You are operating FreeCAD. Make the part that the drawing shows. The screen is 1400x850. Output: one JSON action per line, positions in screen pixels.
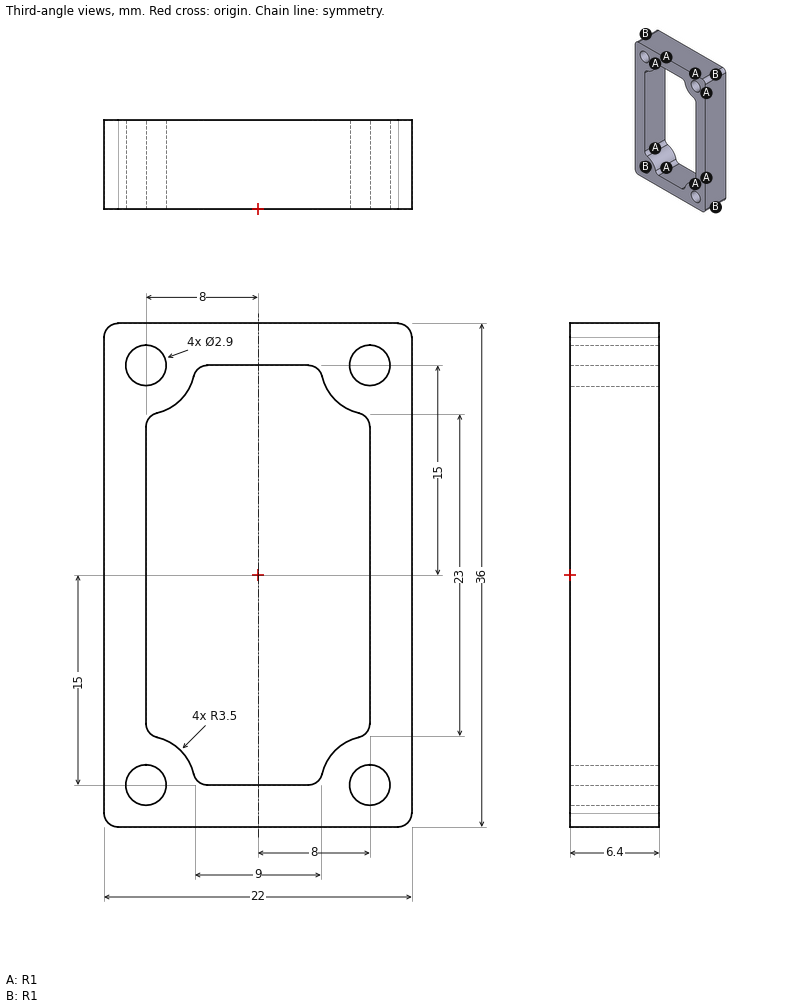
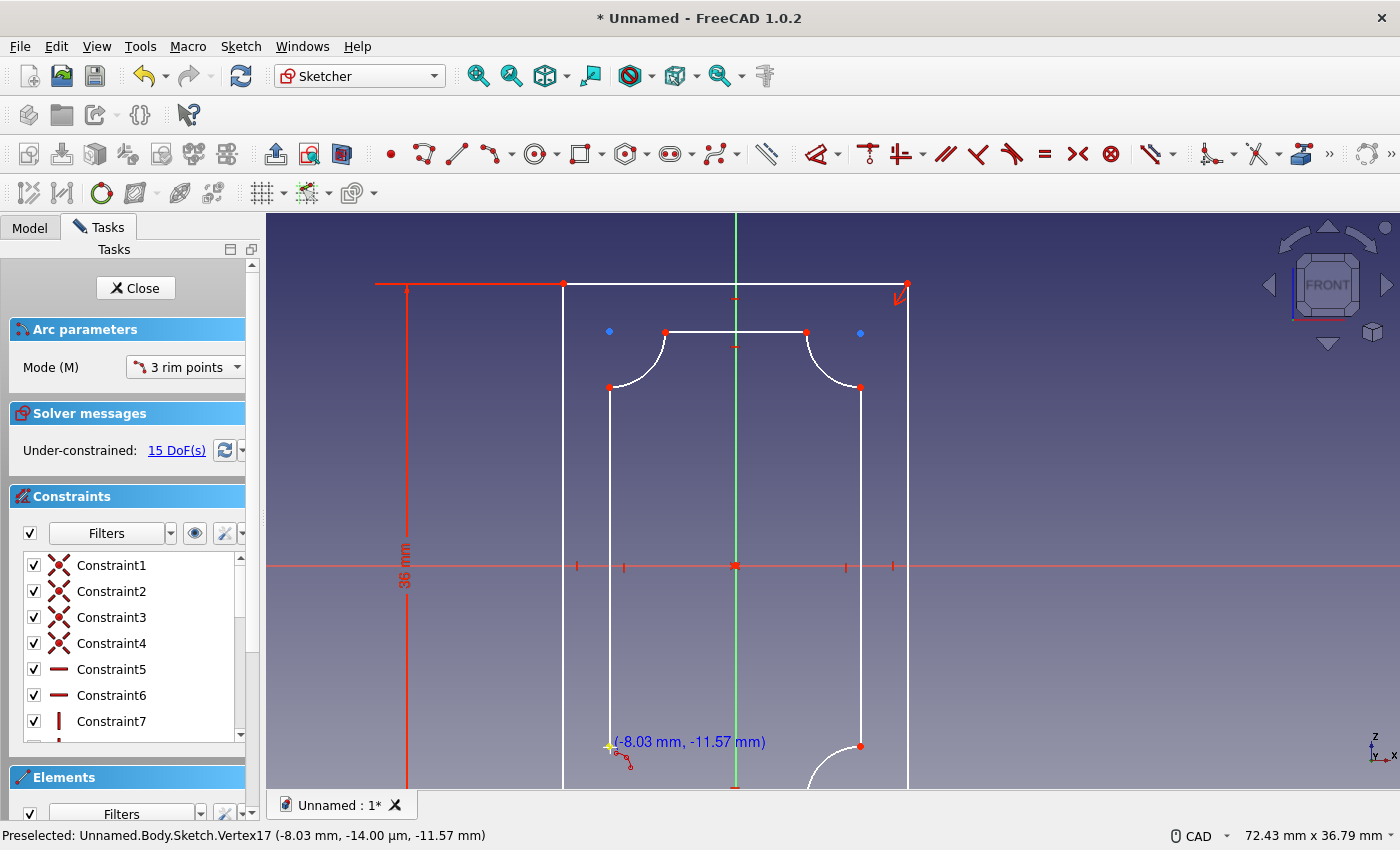
{"action": "scroll", "coordinate": [823, 370], "scroll_direction": "down", "scroll_amount": 2}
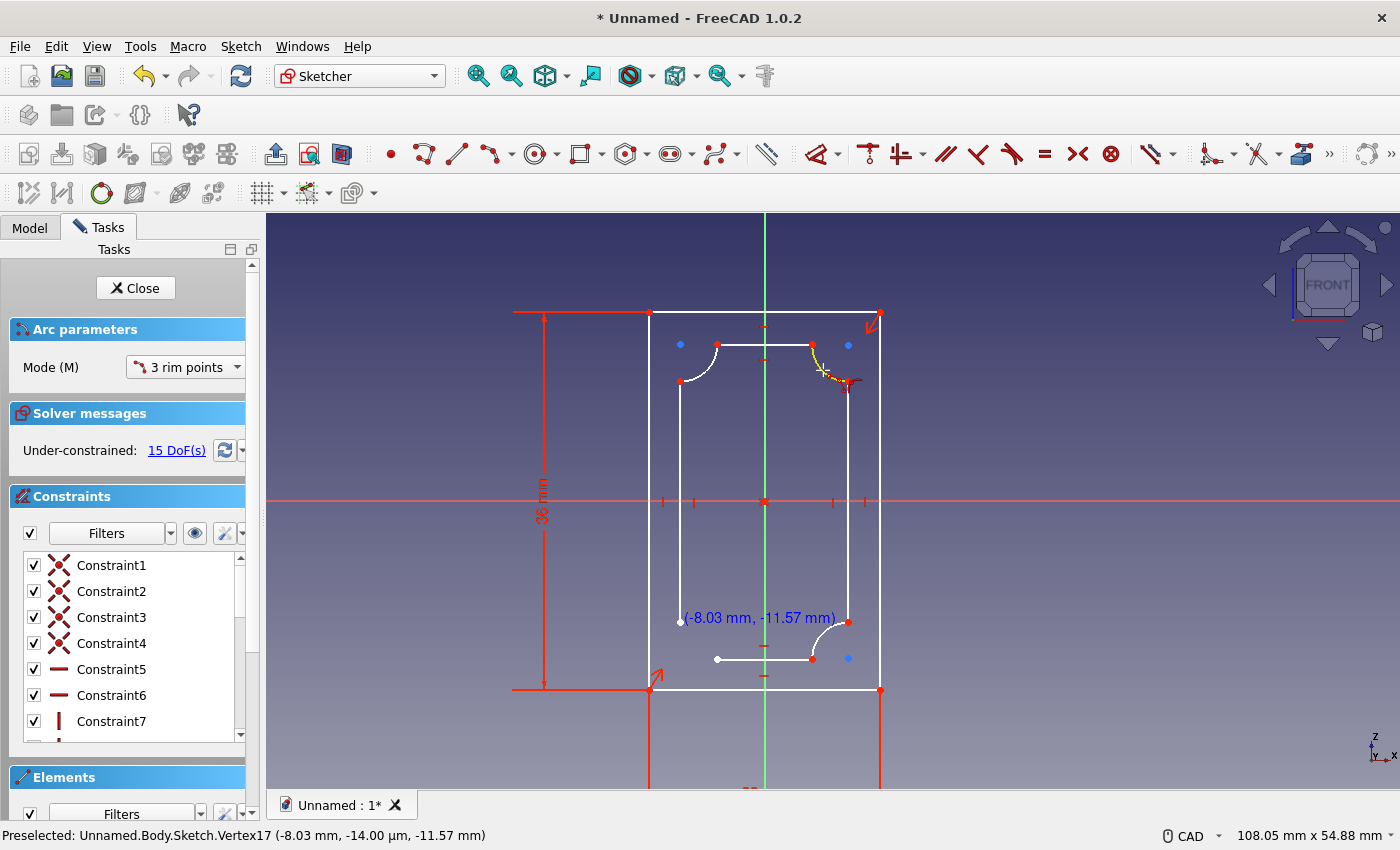
{"action": "left_click", "coordinate": [717, 660]}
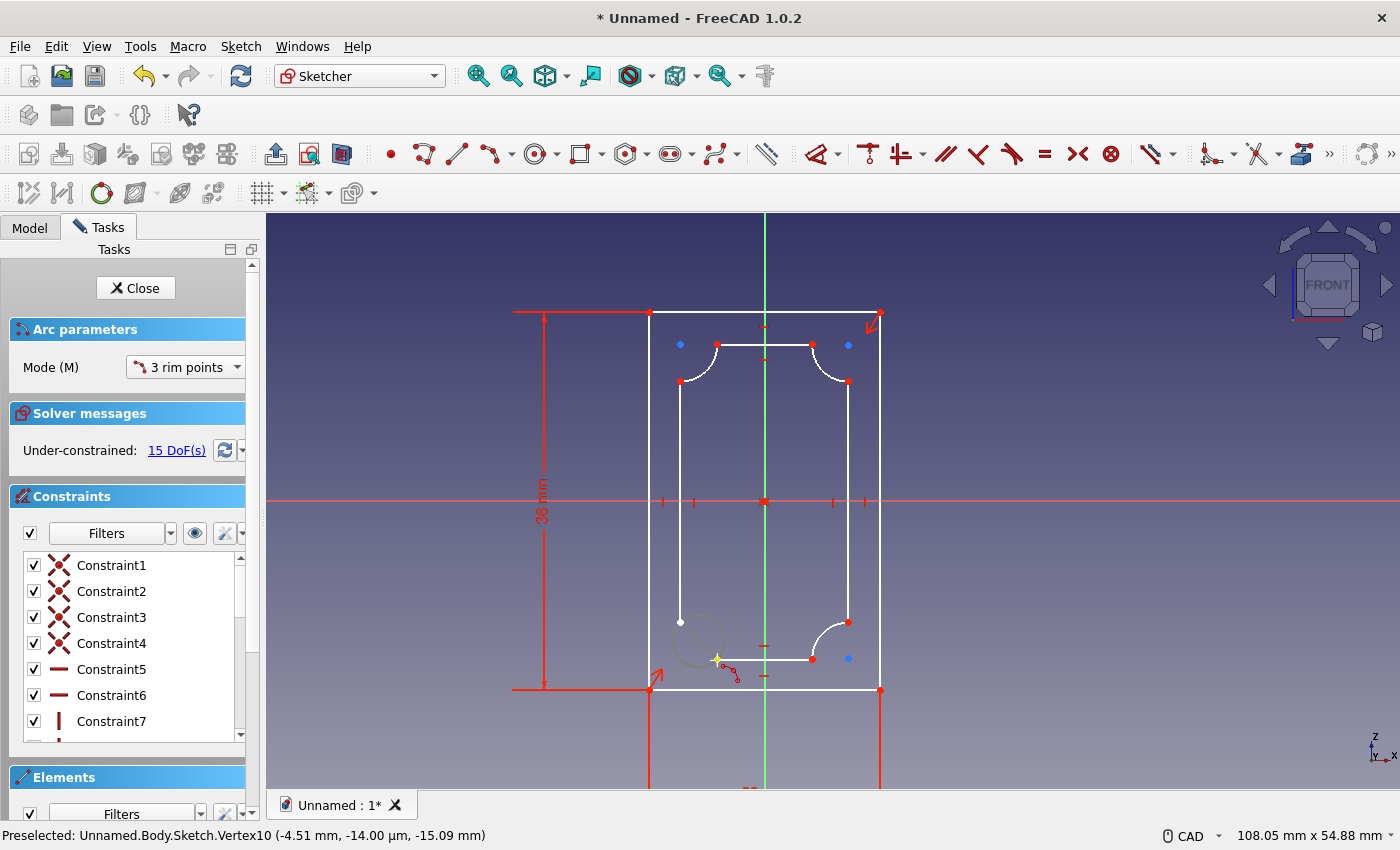
{"action": "scroll", "coordinate": [707, 633], "scroll_direction": "up", "scroll_amount": 2}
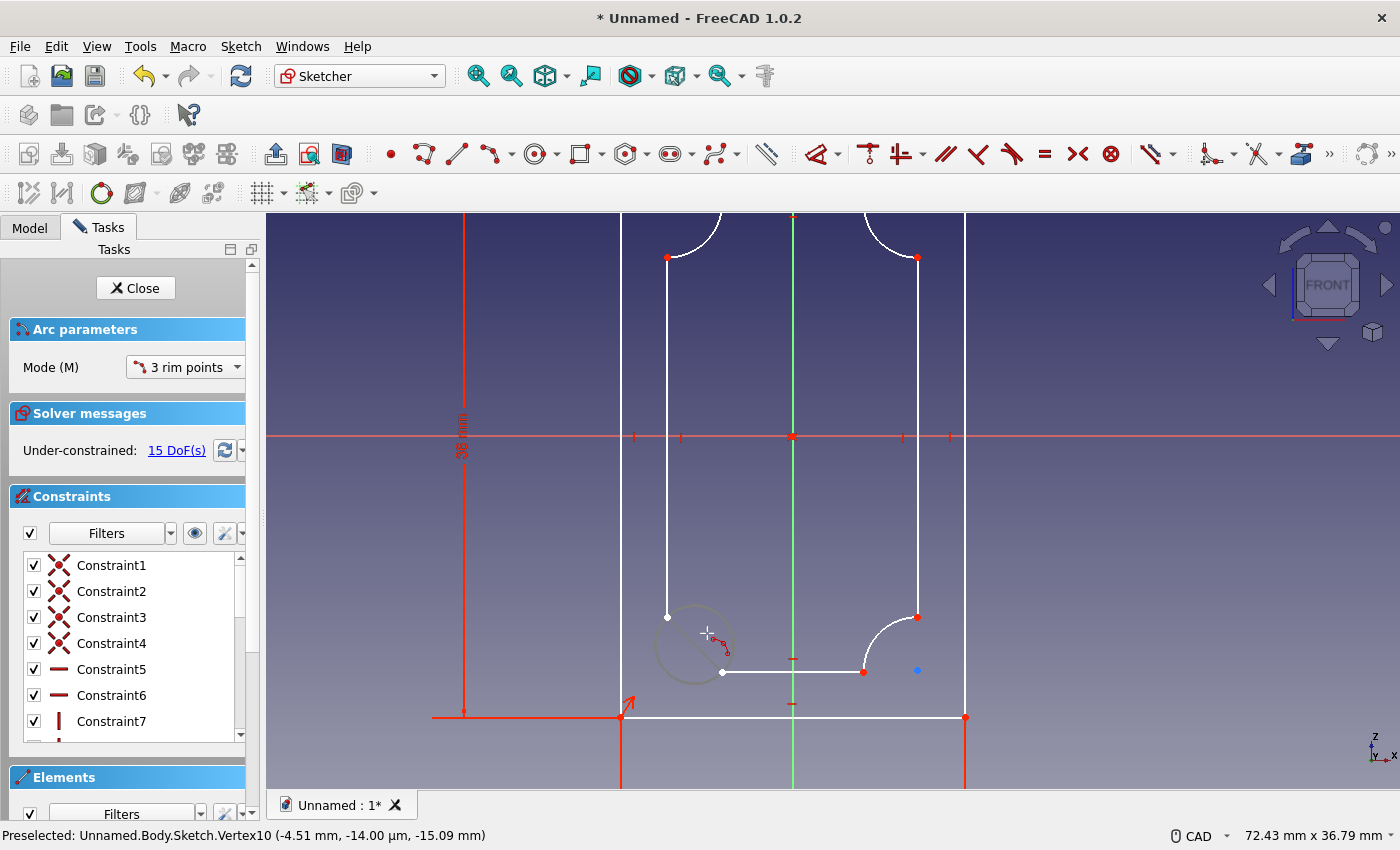
{"action": "left_click", "coordinate": [706, 632]}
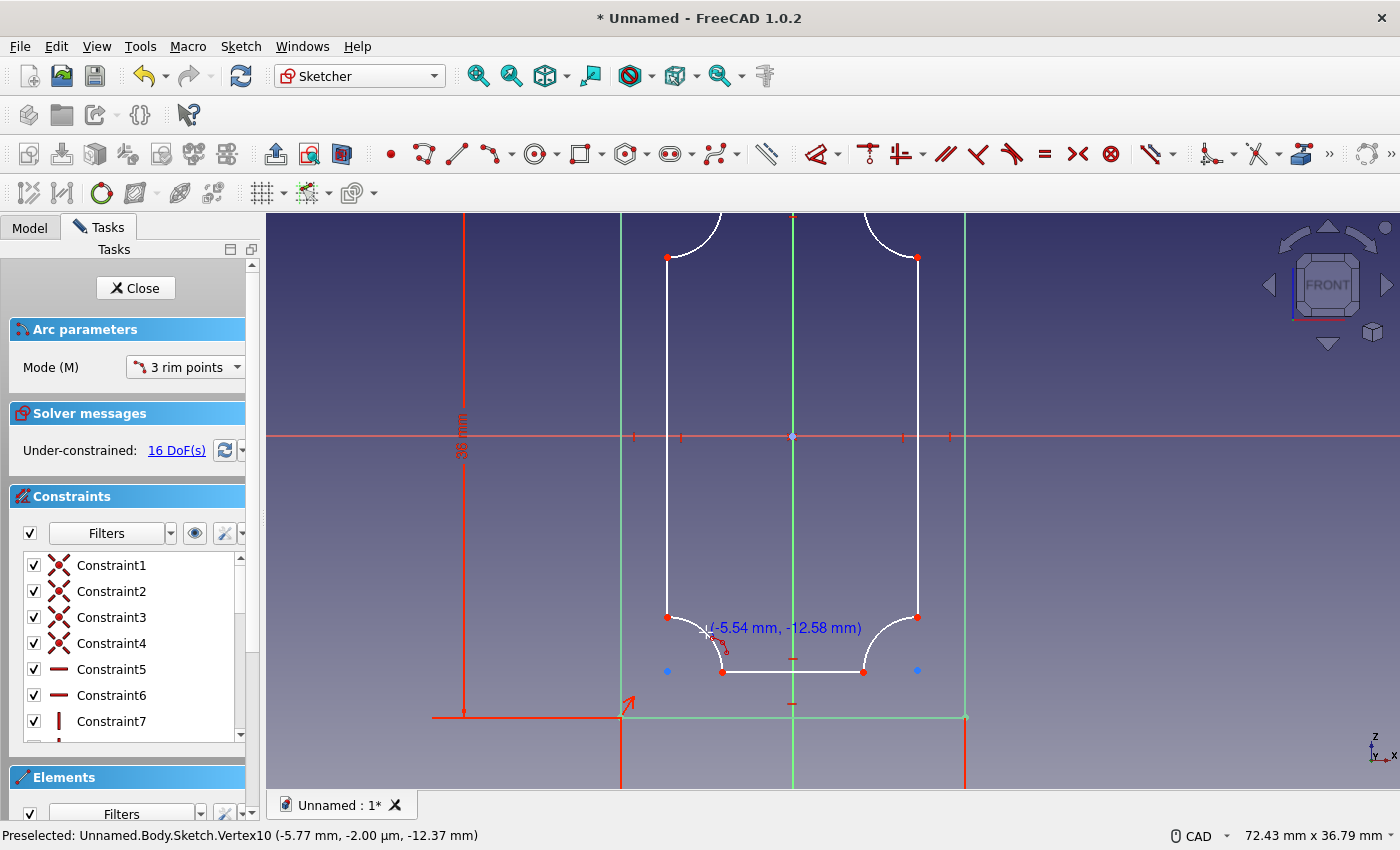
{"action": "left_click", "coordinate": [534, 154]}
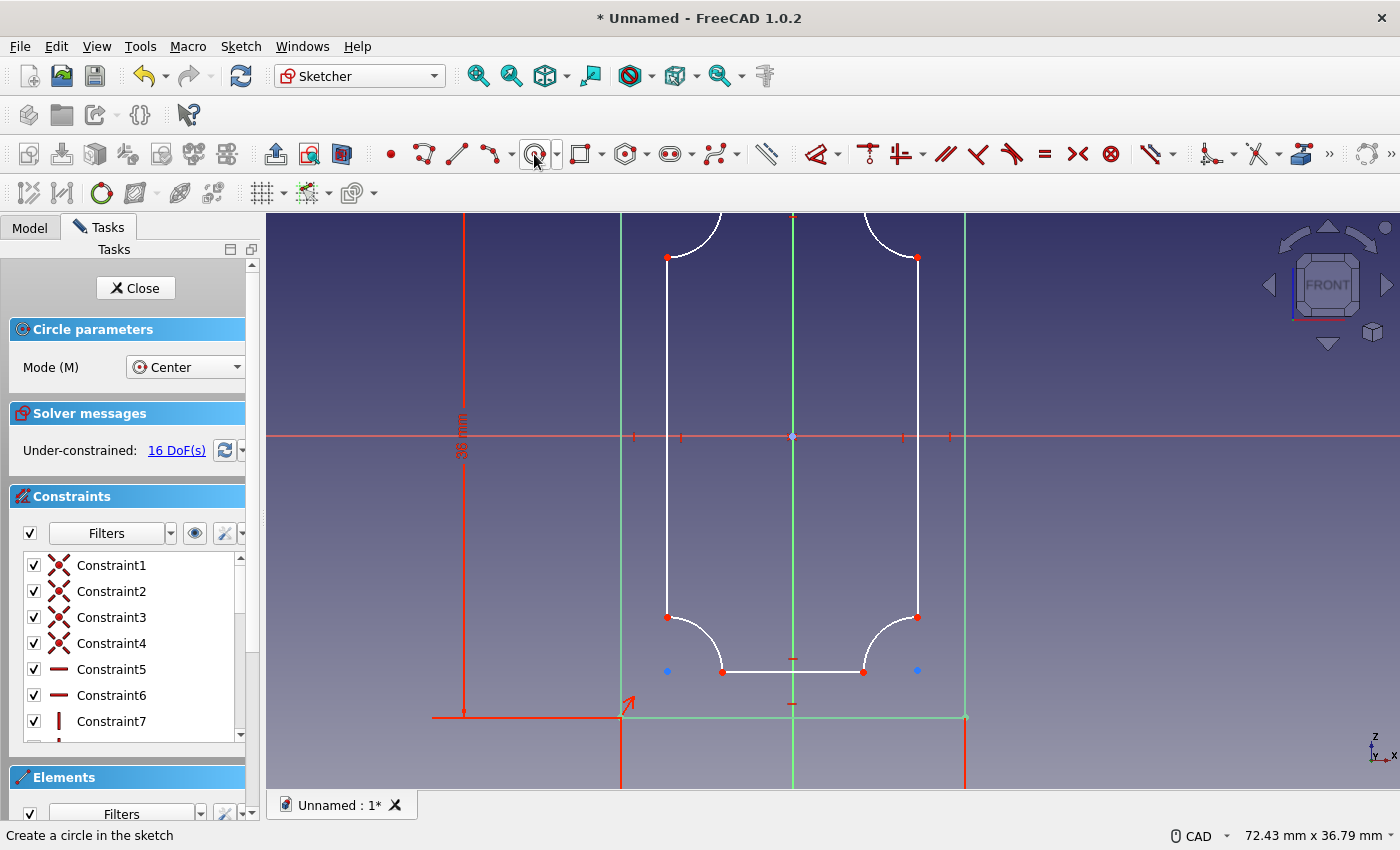
{"action": "scroll", "coordinate": [707, 633], "scroll_direction": "down", "scroll_amount": 2}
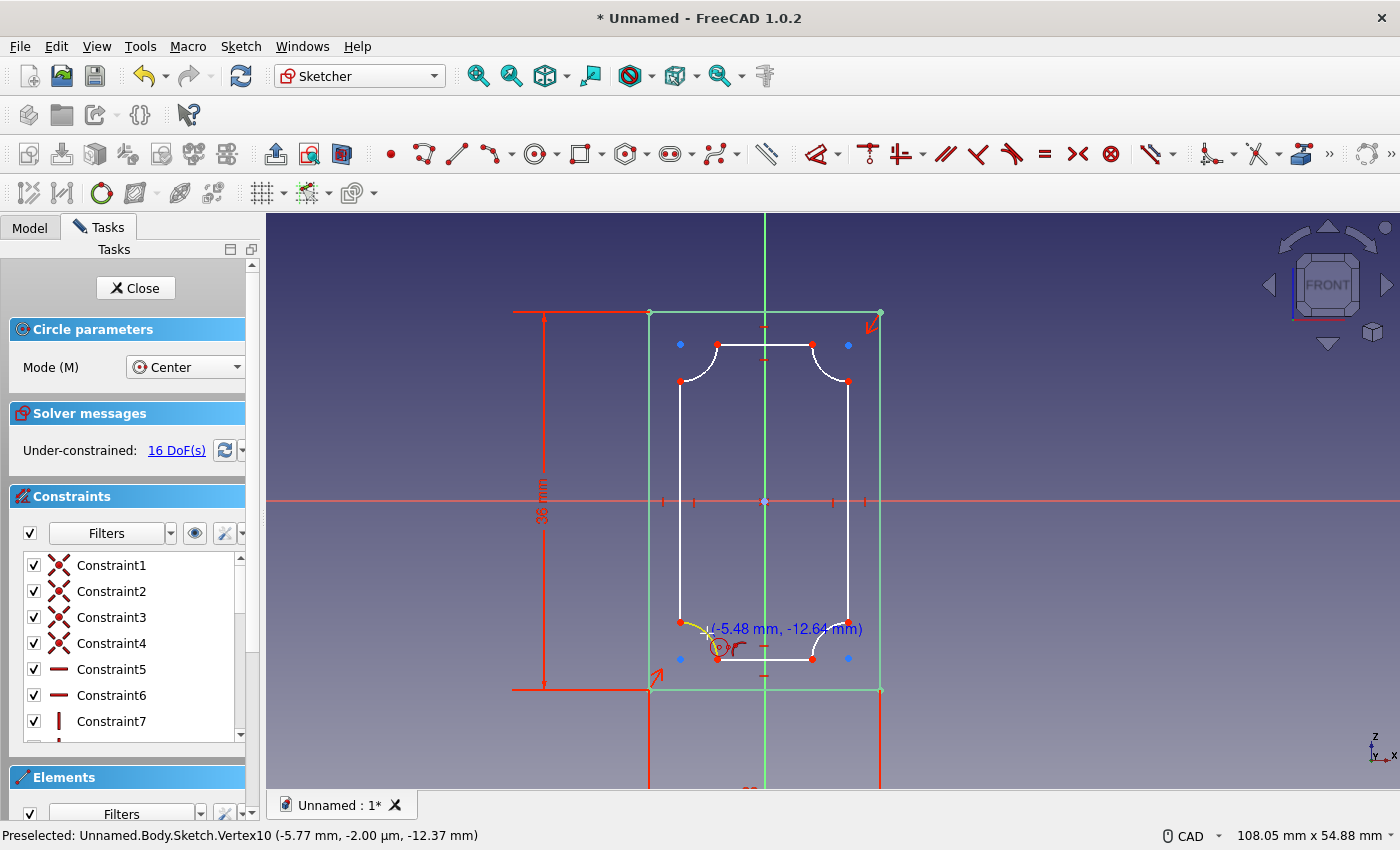
{"action": "scroll", "coordinate": [681, 344], "scroll_direction": "up", "scroll_amount": 2}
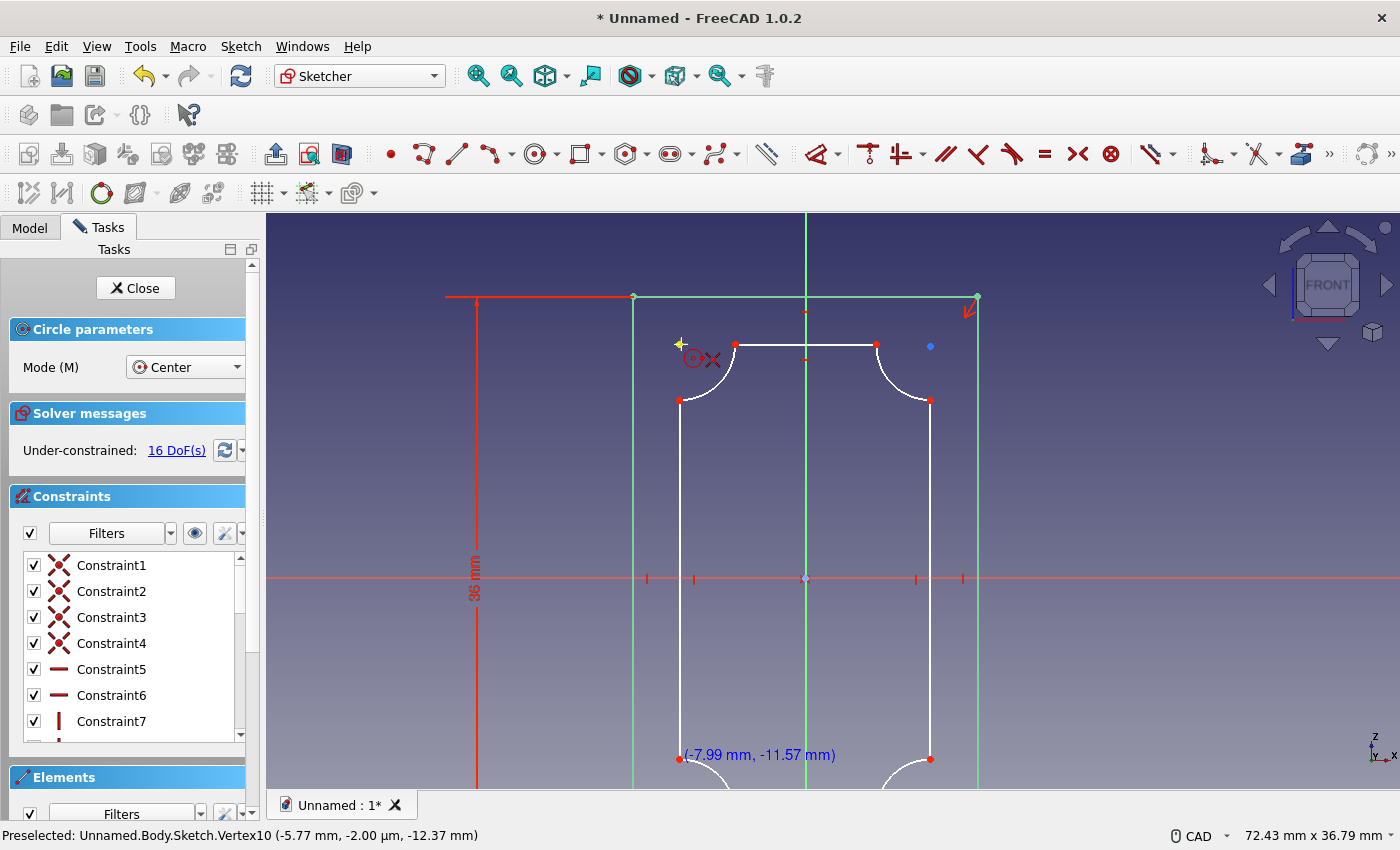
{"action": "left_click", "coordinate": [680, 344]}
{"action": "mouse_move", "coordinate": [696, 328]}